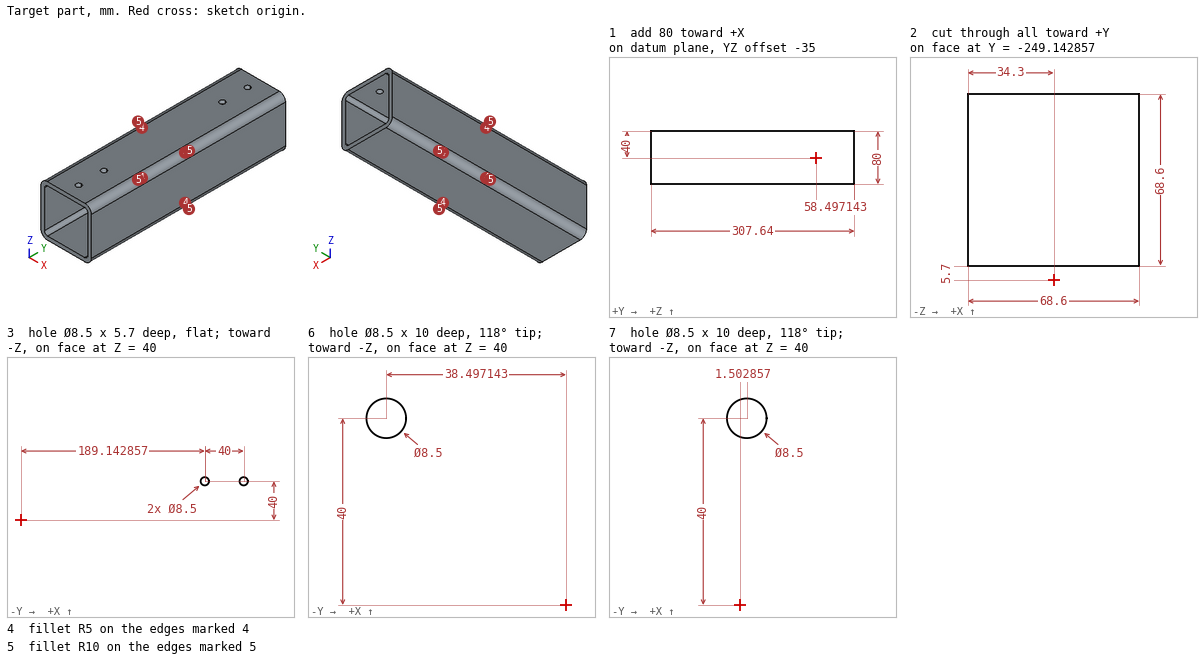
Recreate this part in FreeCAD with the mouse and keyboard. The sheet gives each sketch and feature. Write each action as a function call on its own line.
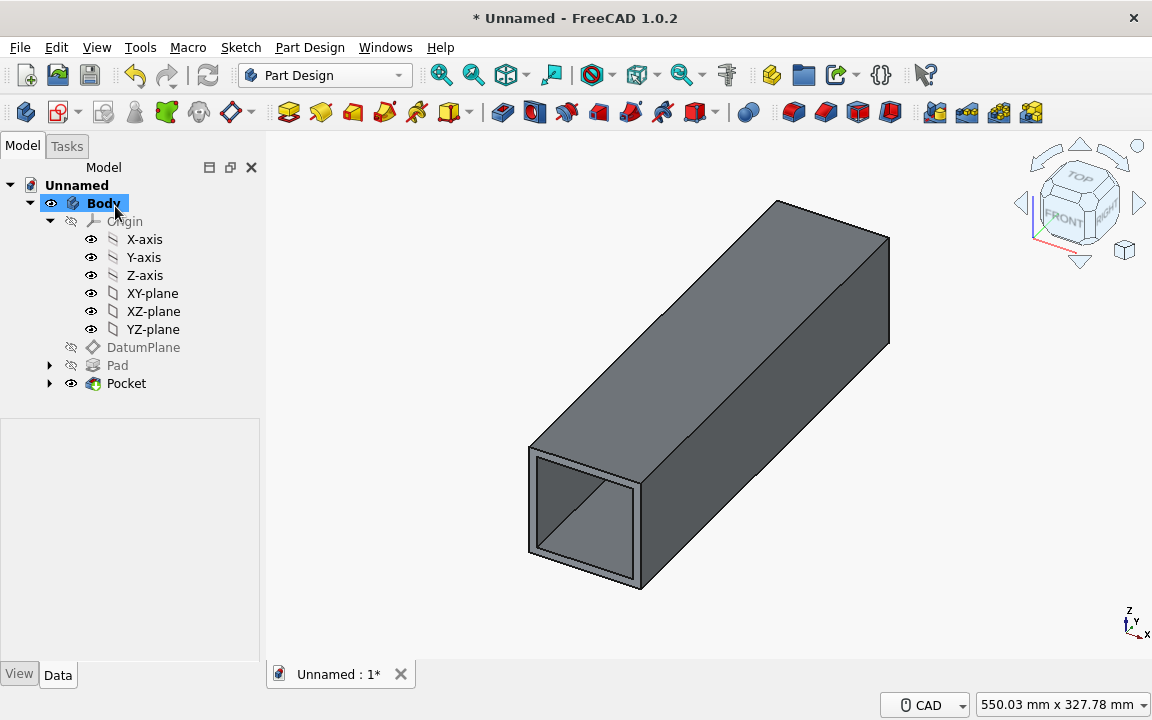
click(744, 306)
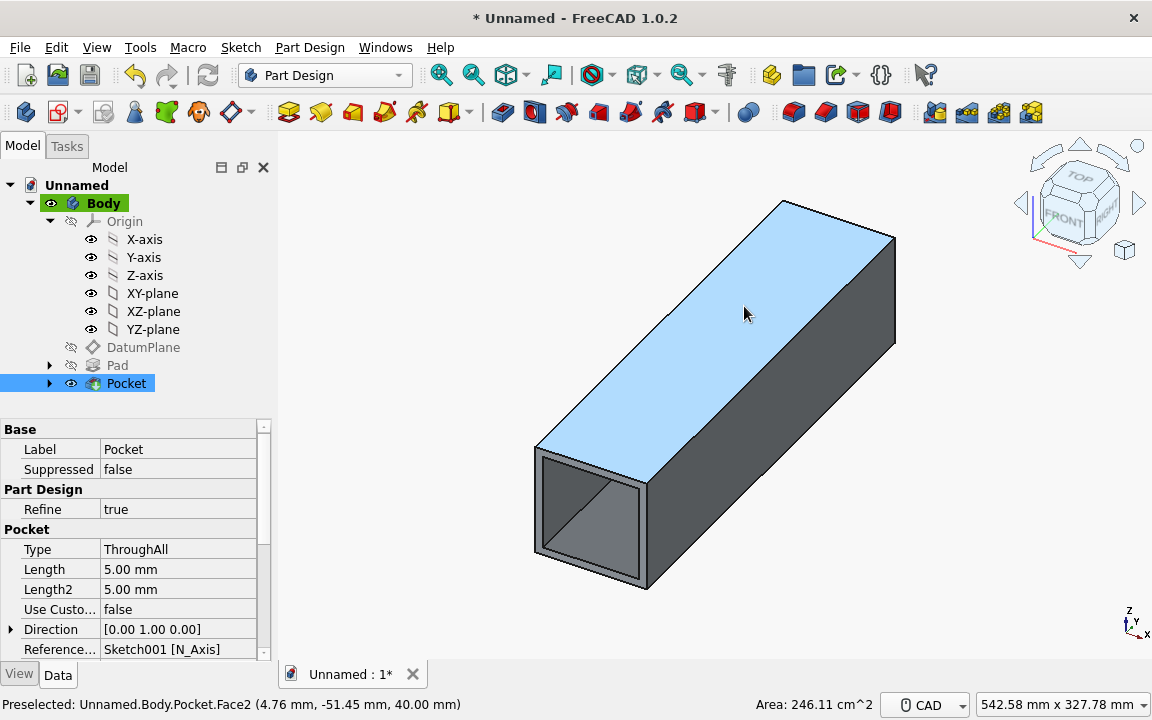
click(58, 112)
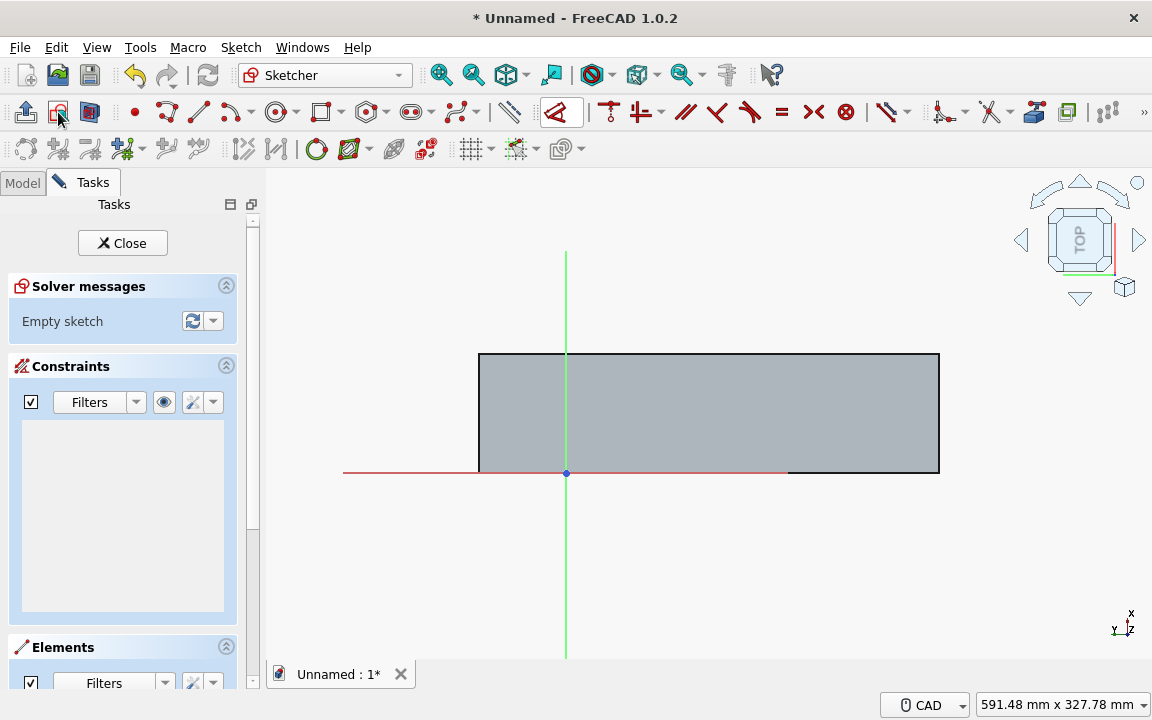
scroll(917, 413, up, 10)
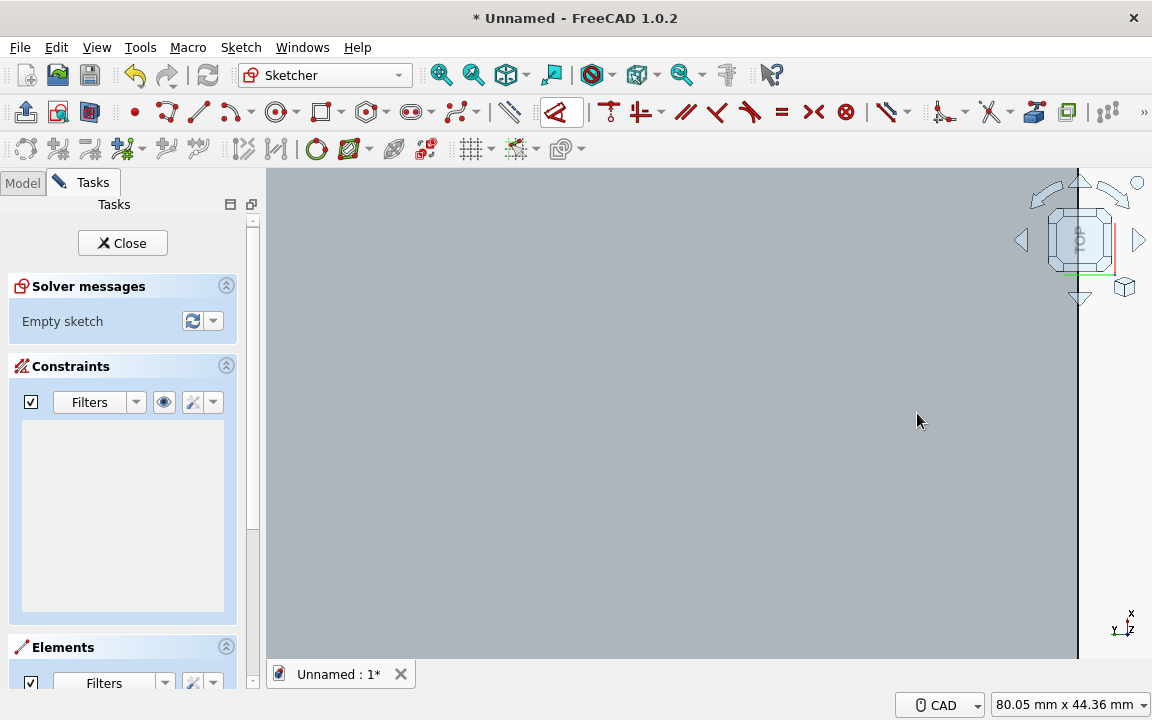
click(276, 112)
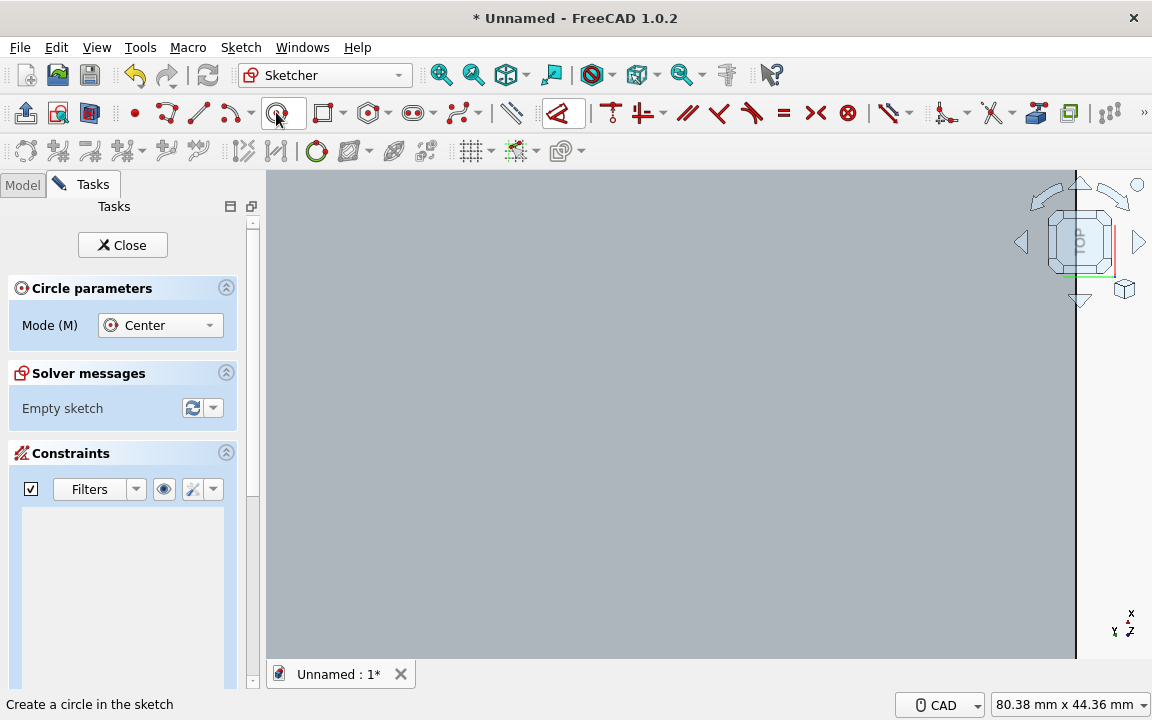
click(415, 414)
move(448, 381)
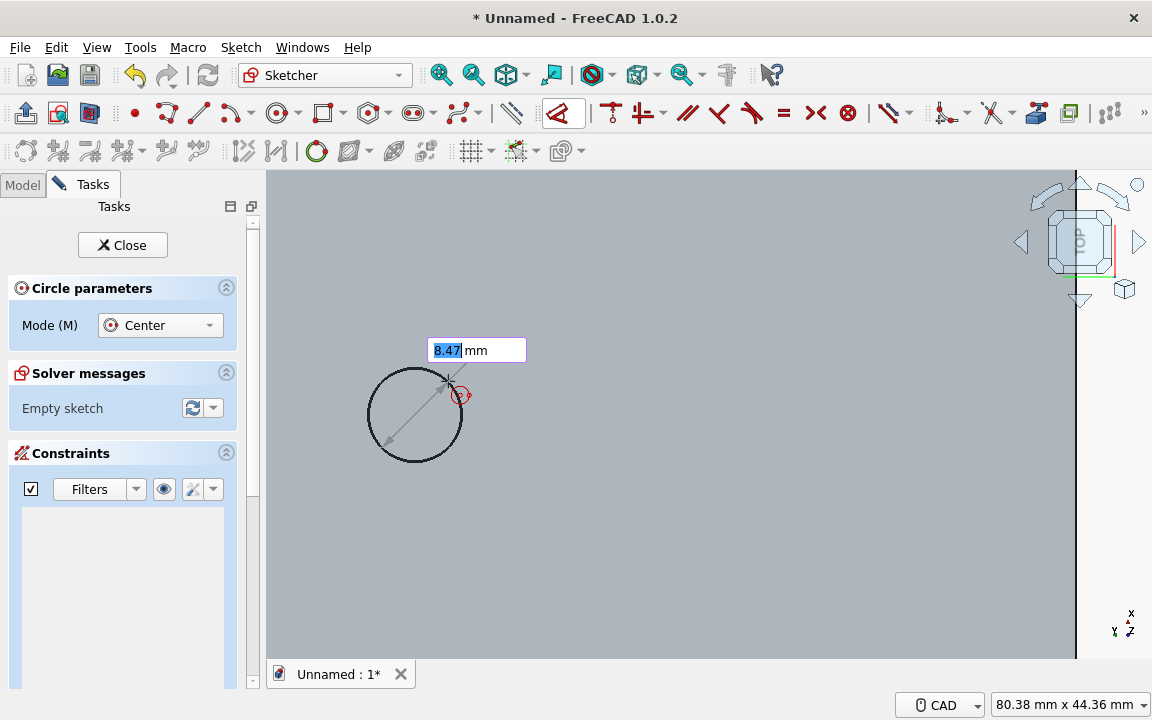
text(8.5)
key(Return)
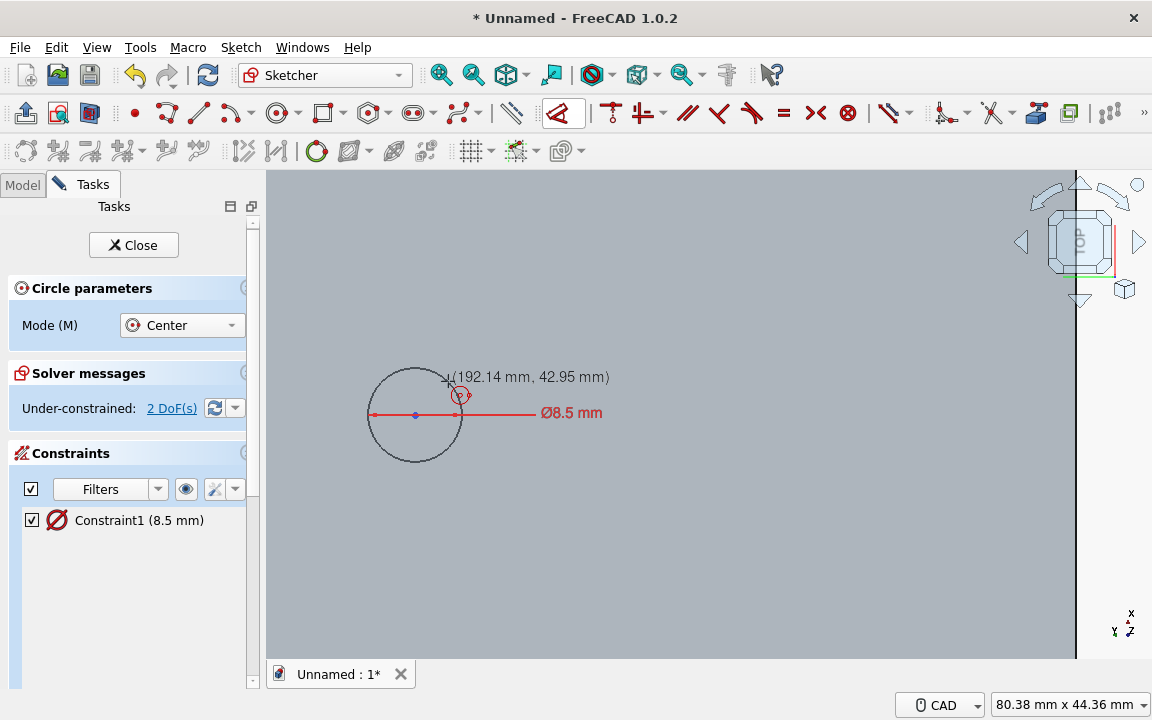
click(856, 414)
move(889, 381)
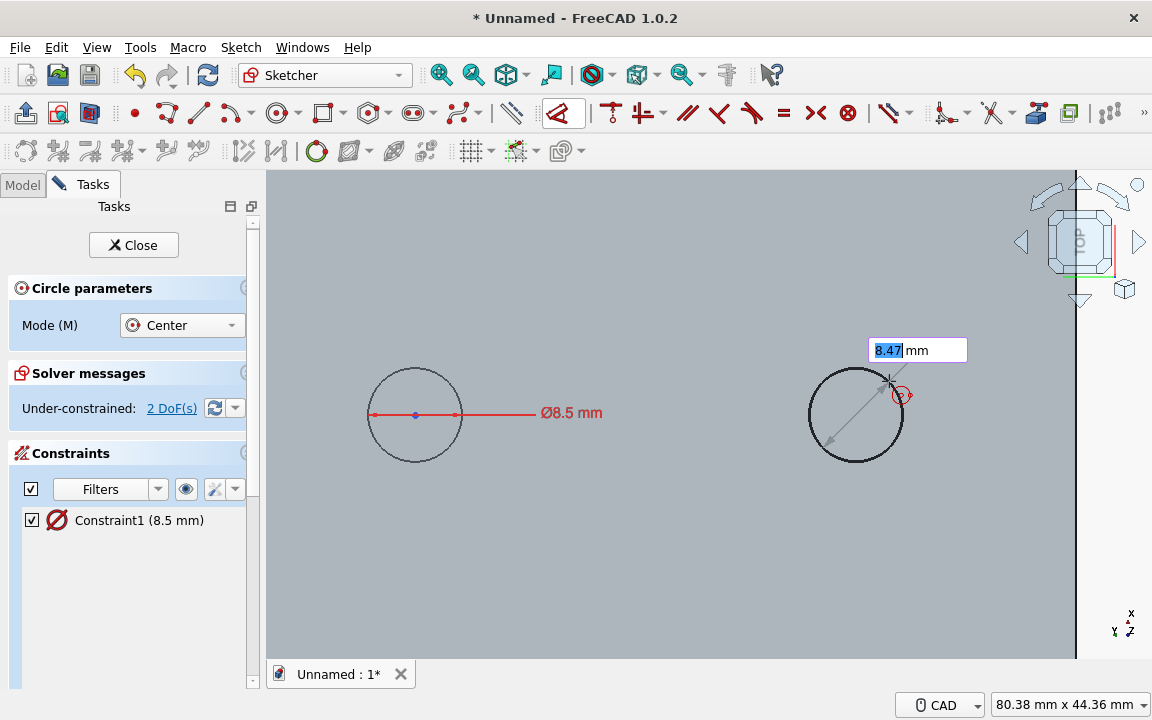
text(8.5)
key(Return)
key(Escape)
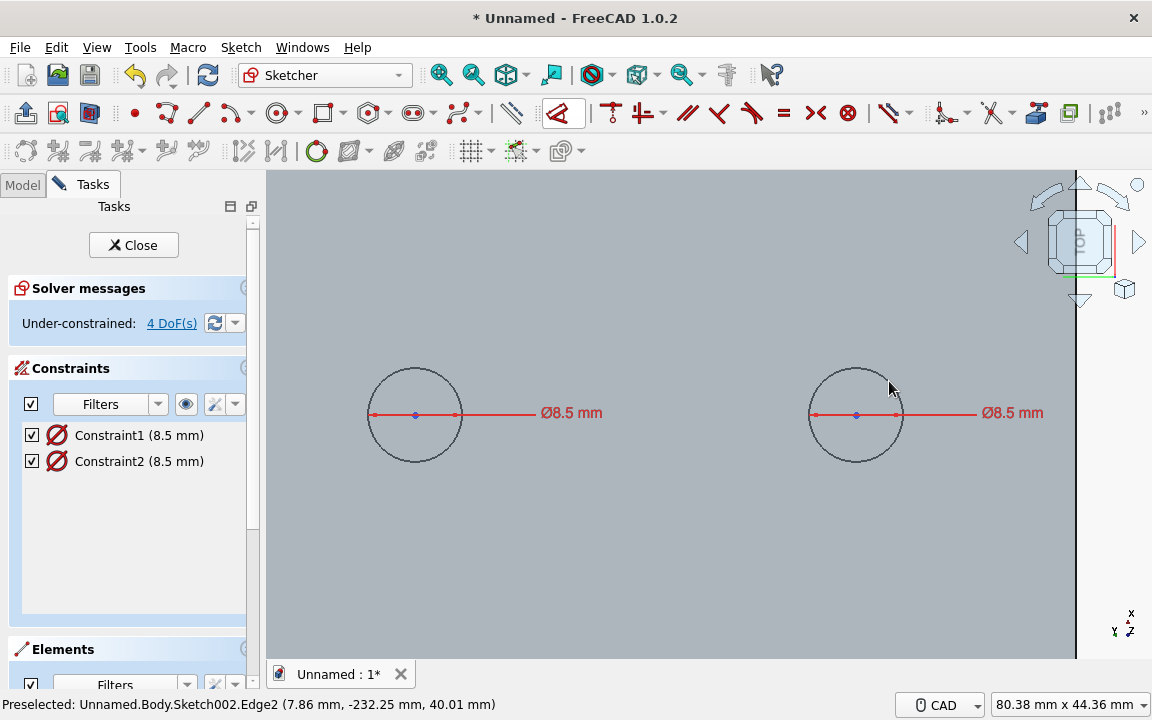
click(415, 415)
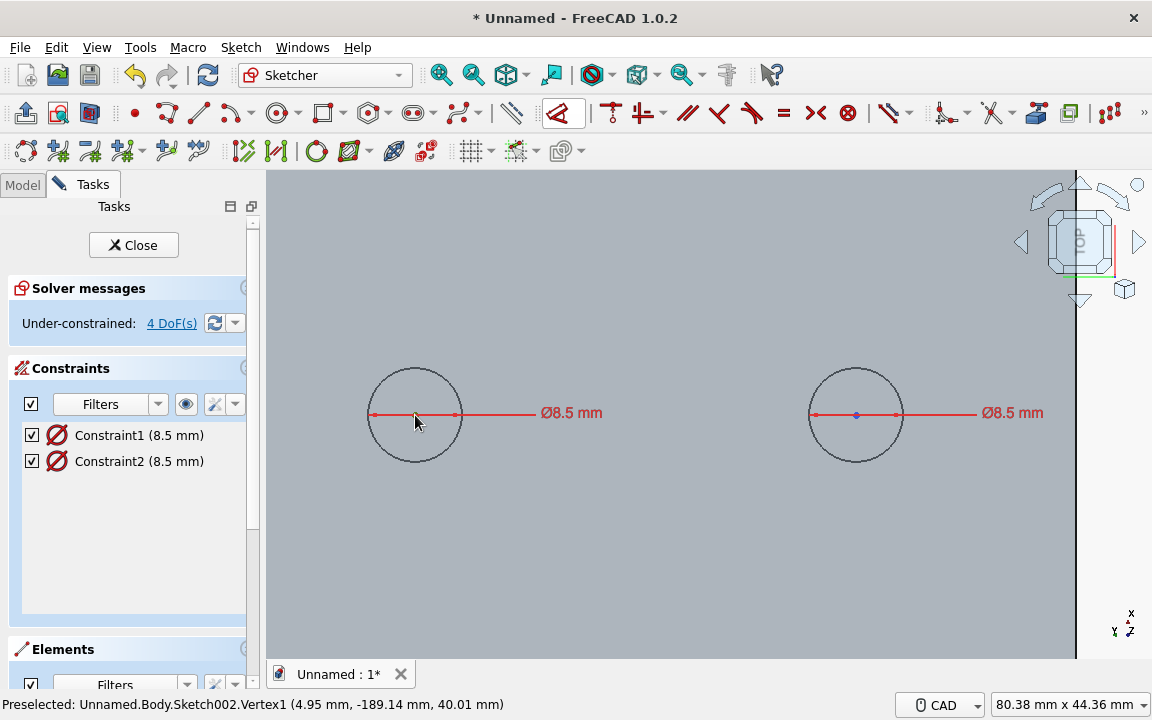
click(856, 415)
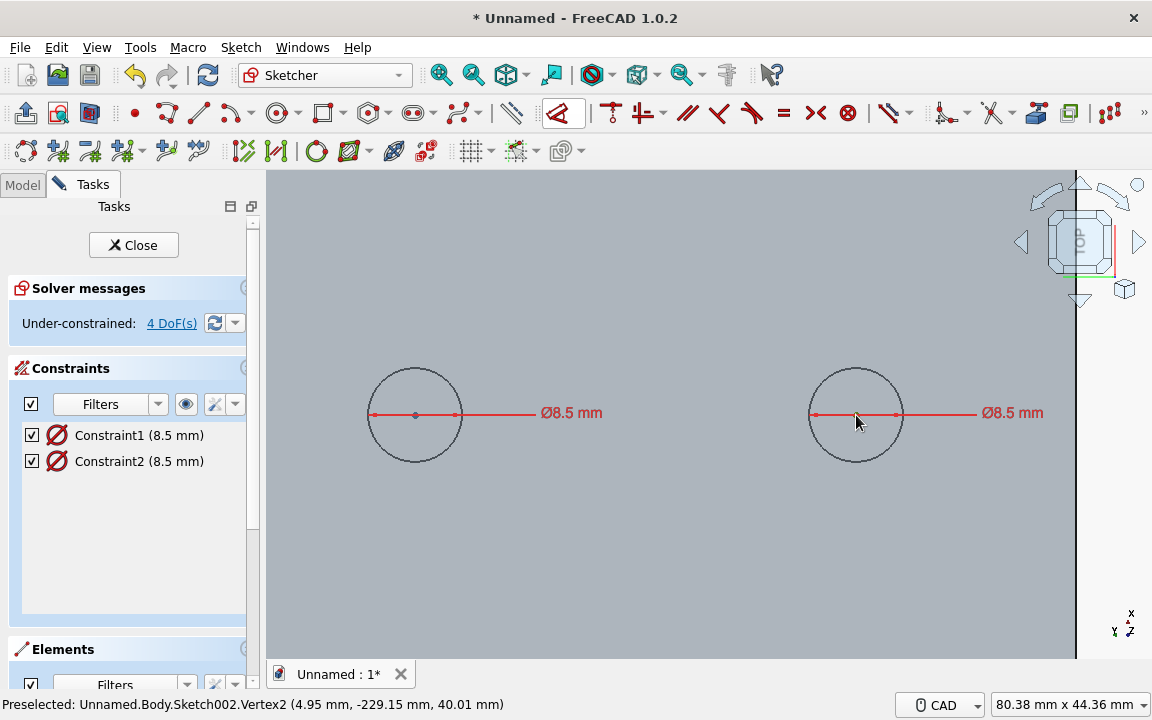
key(h)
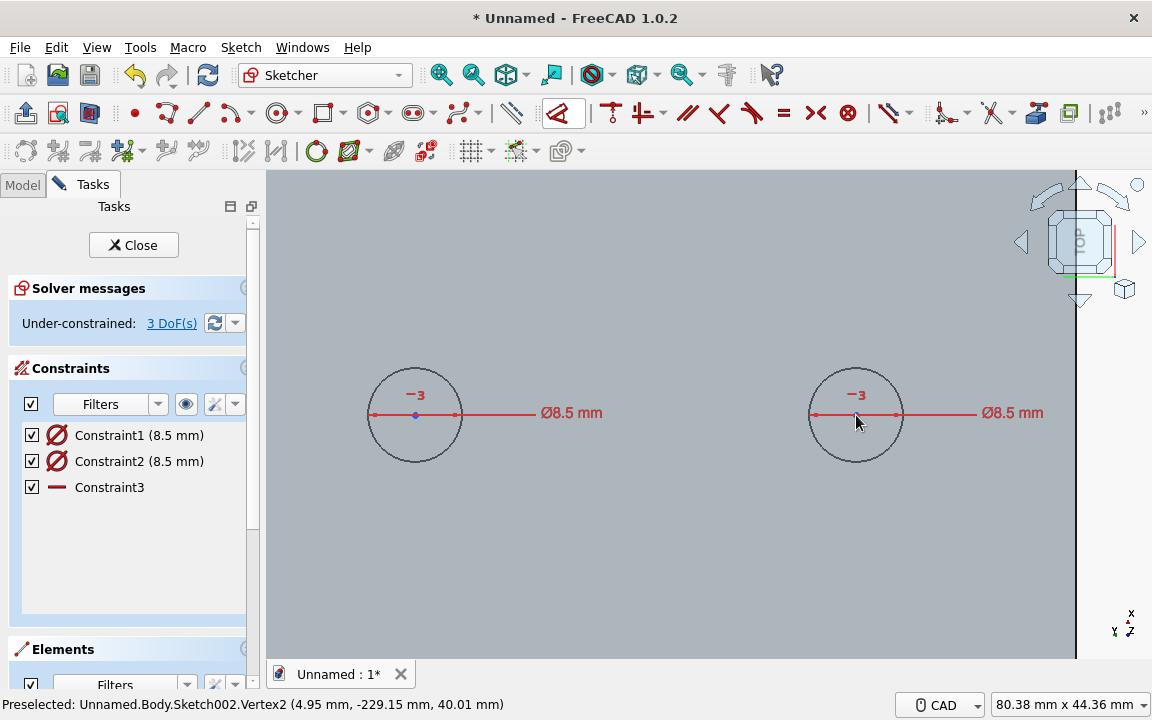
click(415, 415)